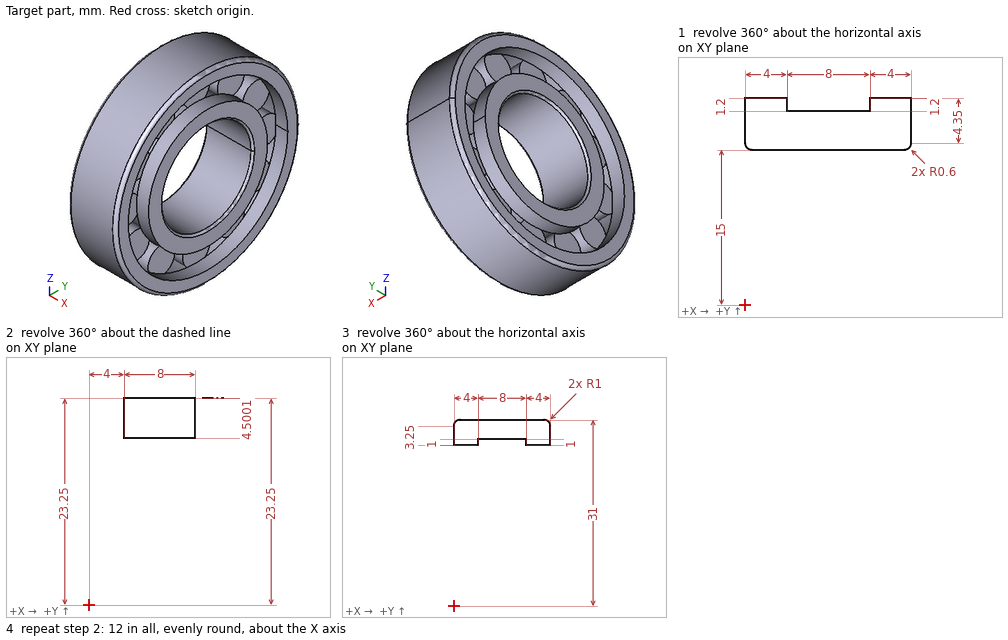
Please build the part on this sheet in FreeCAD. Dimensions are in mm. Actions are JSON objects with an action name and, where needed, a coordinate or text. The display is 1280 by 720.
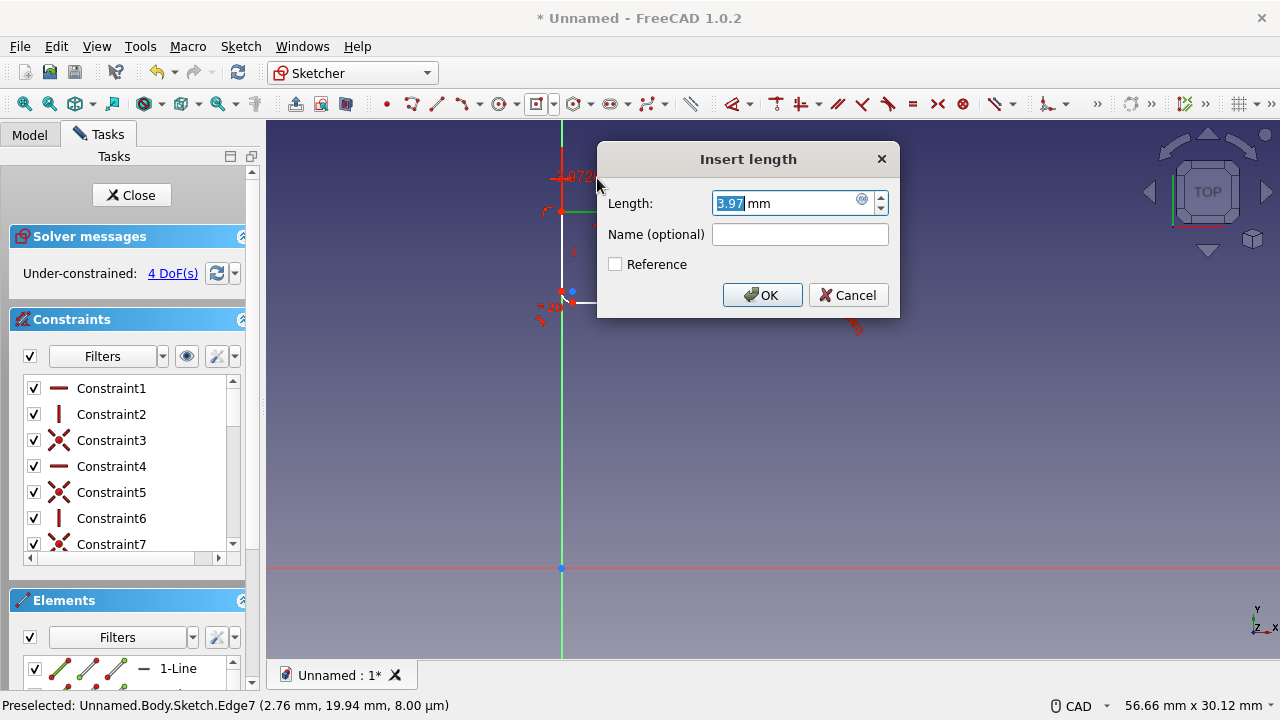
{"action": "type", "text": "4"}
{"action": "key", "text": "Return"}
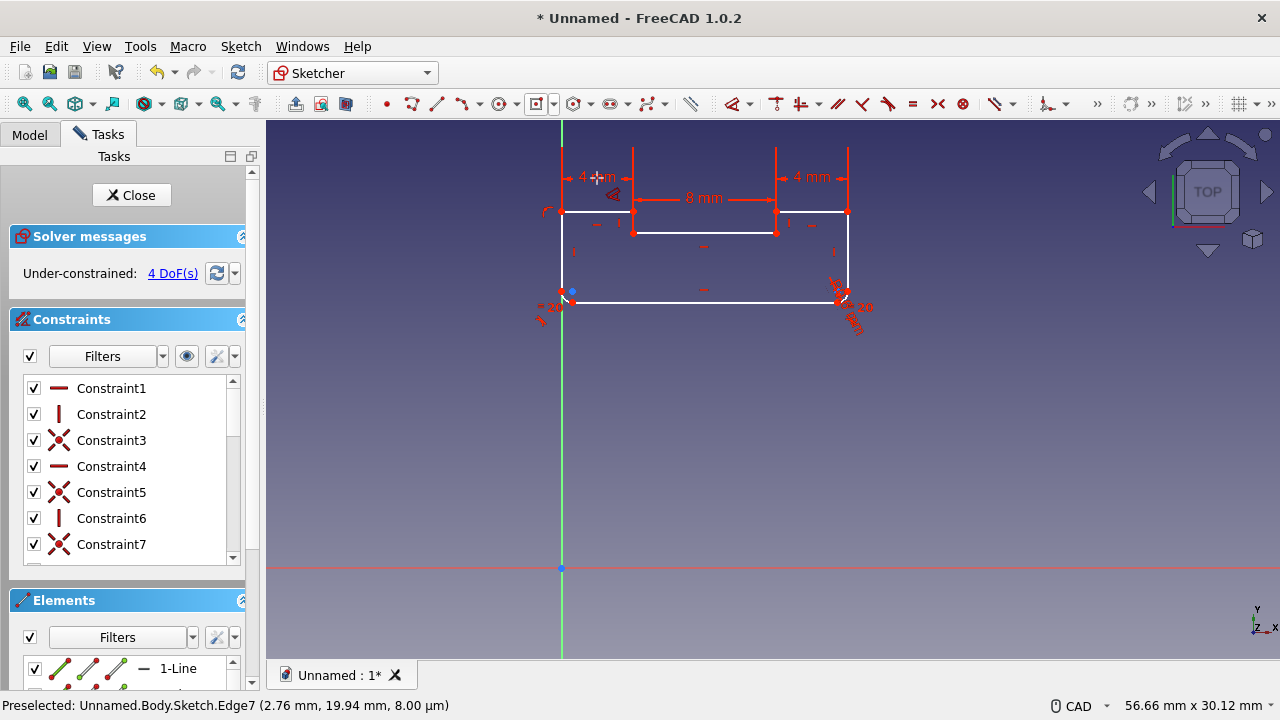
{"action": "scroll", "coordinate": [776, 223], "scroll_direction": "up", "scroll_amount": 4}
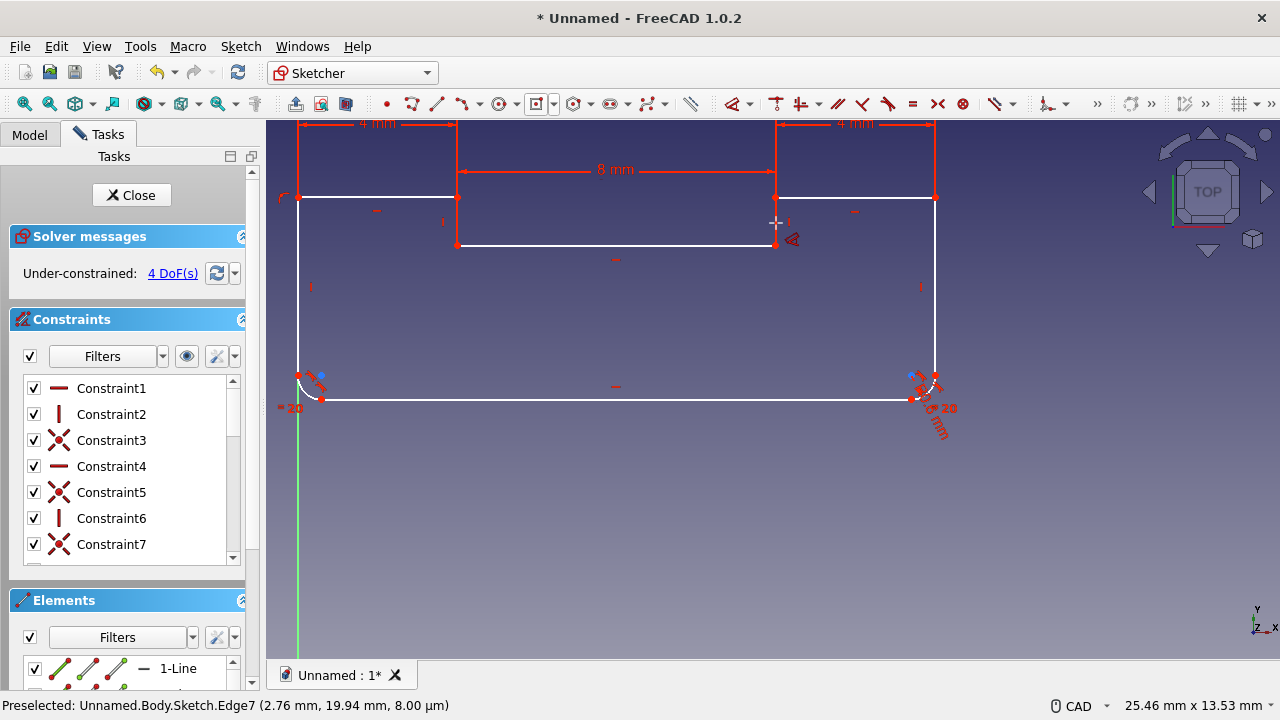
{"action": "left_click", "coordinate": [776, 222]}
{"action": "left_click", "coordinate": [810, 222]}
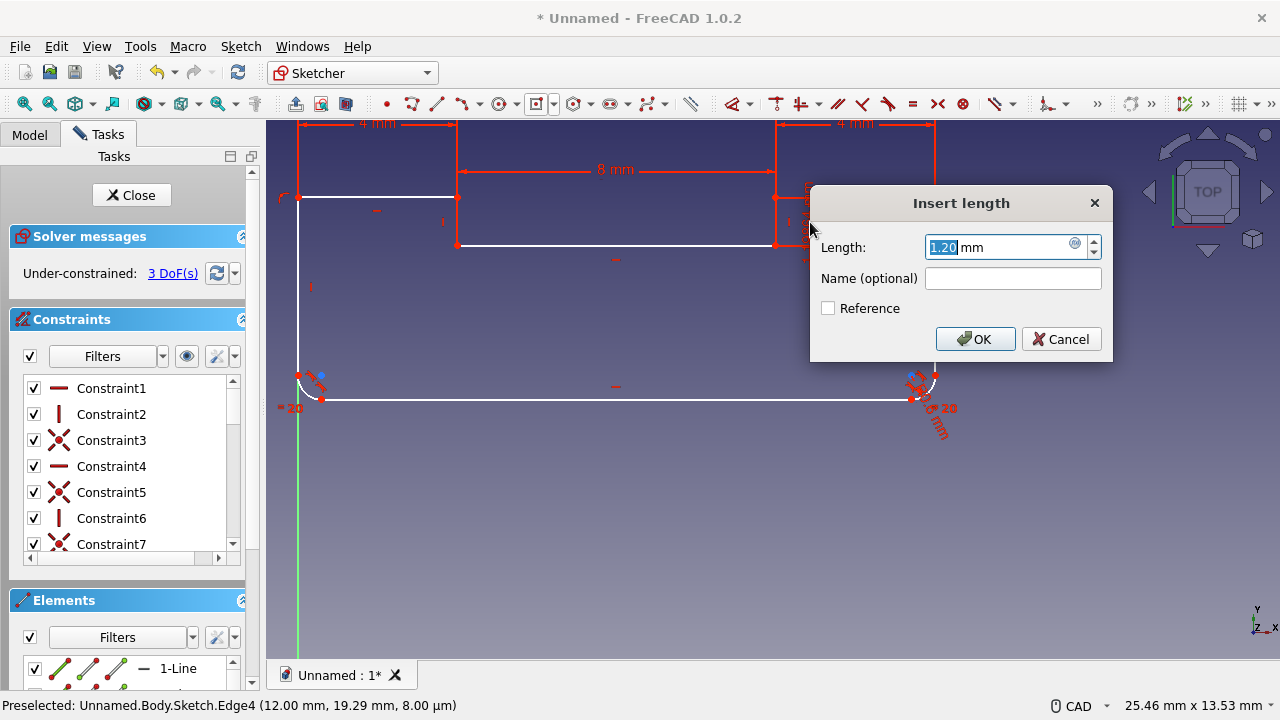
{"action": "type", "text": "1.2"}
{"action": "key", "text": "Return"}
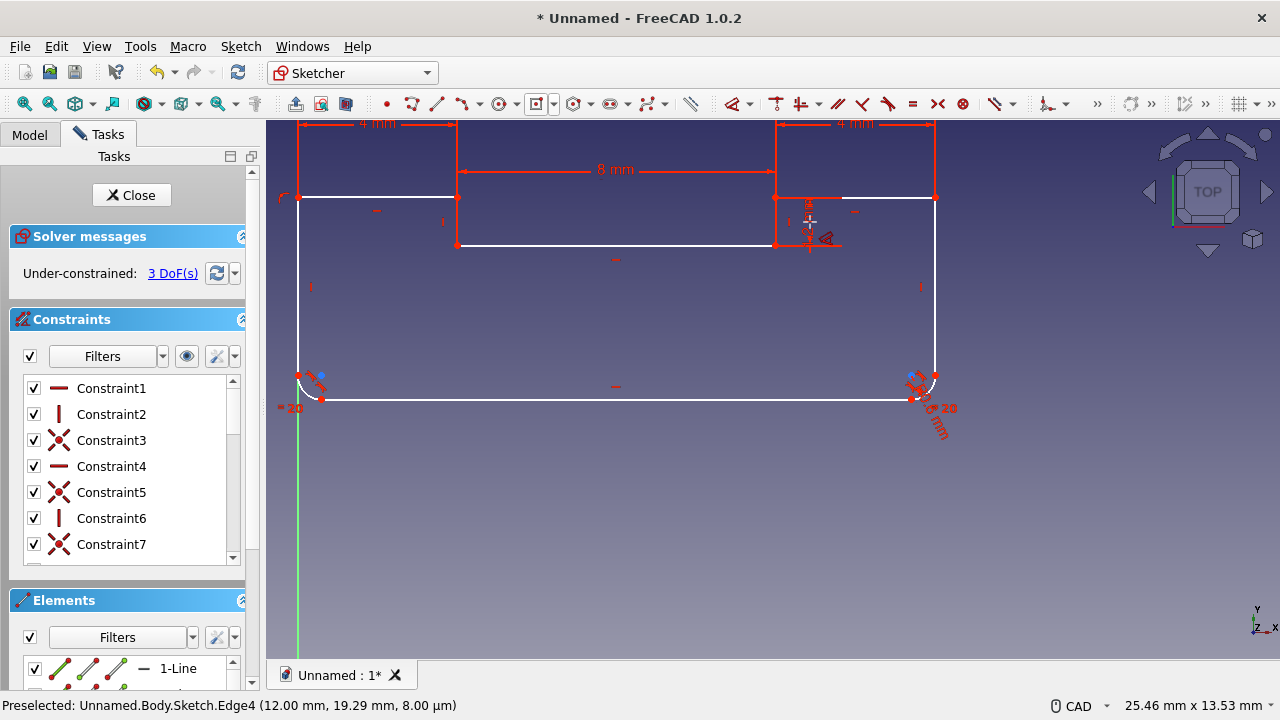
{"action": "left_click", "coordinate": [457, 231]}
{"action": "left_click", "coordinate": [423, 221]}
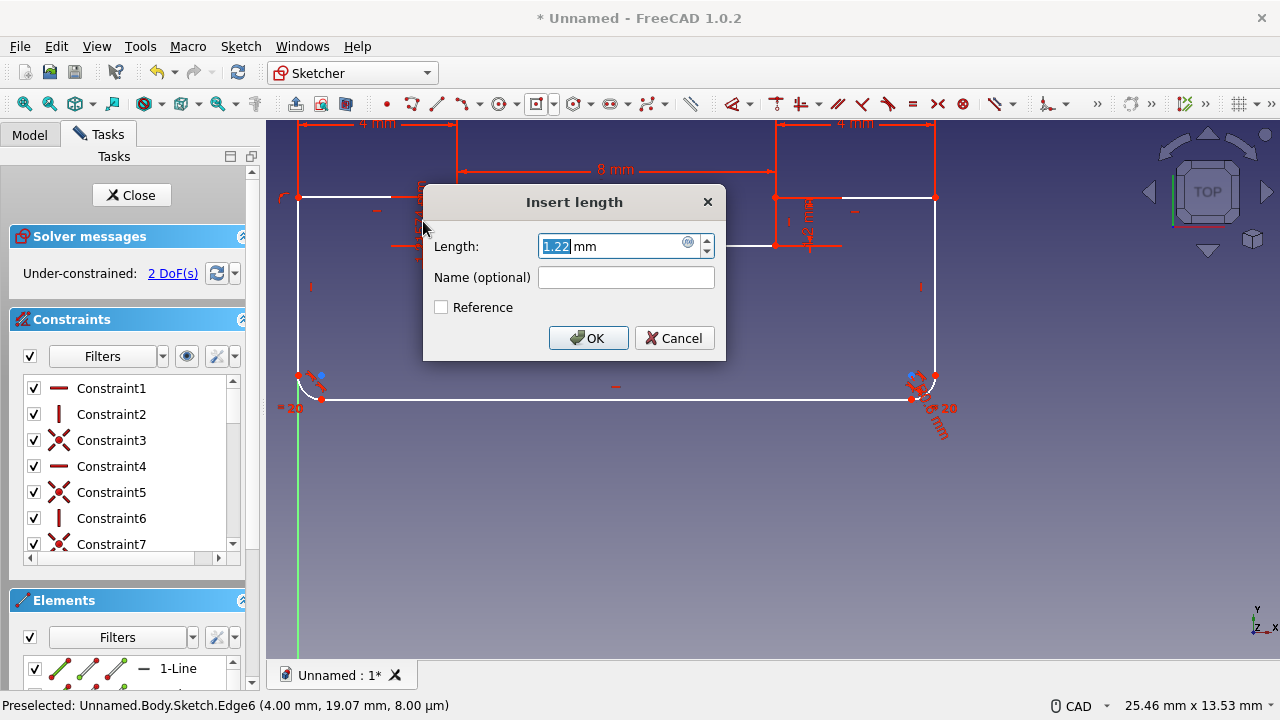
{"action": "type", "text": "1.2"}
{"action": "key", "text": "Return"}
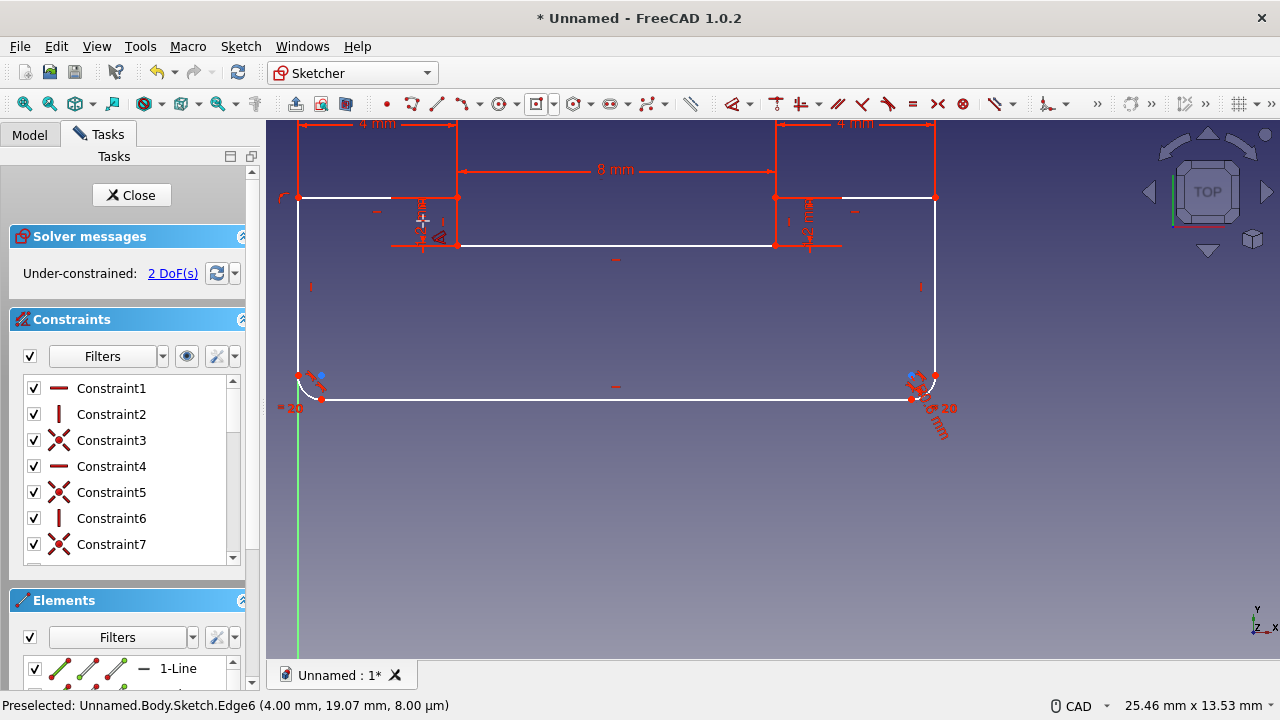
{"action": "left_click", "coordinate": [322, 400]}
{"action": "left_click", "coordinate": [356, 515]}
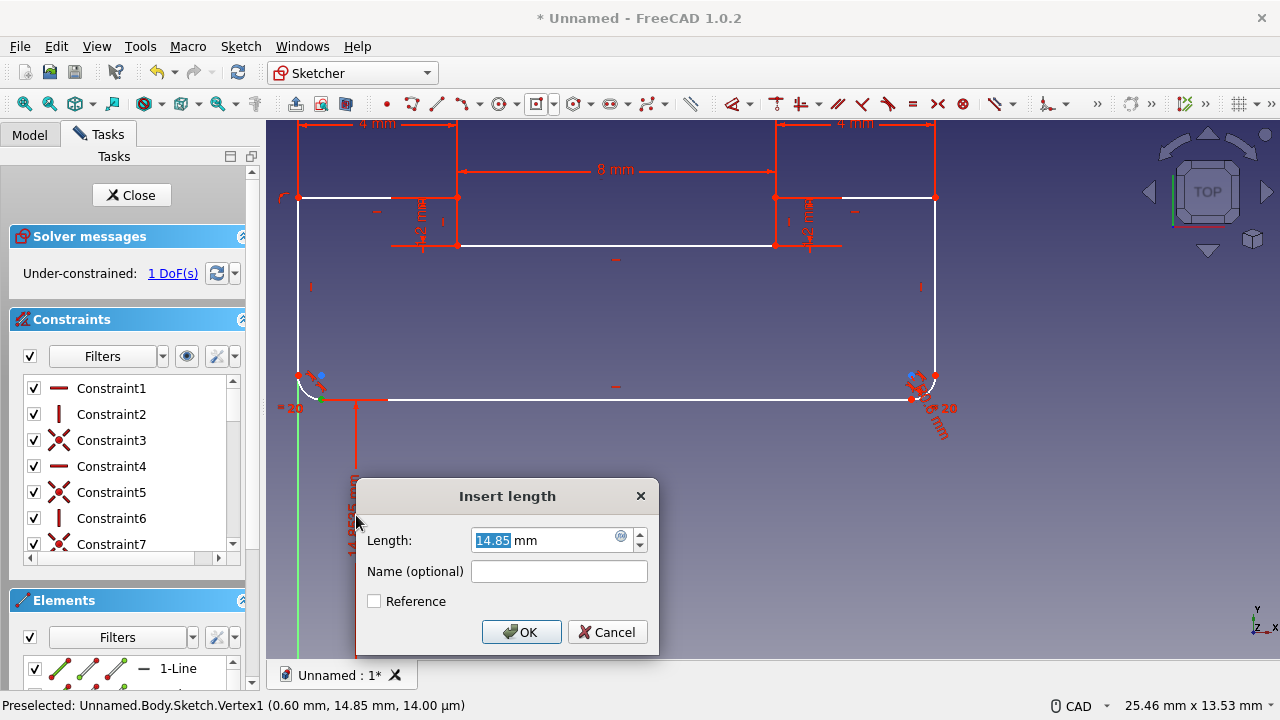
{"action": "type", "text": "15"}
{"action": "key", "text": "Return"}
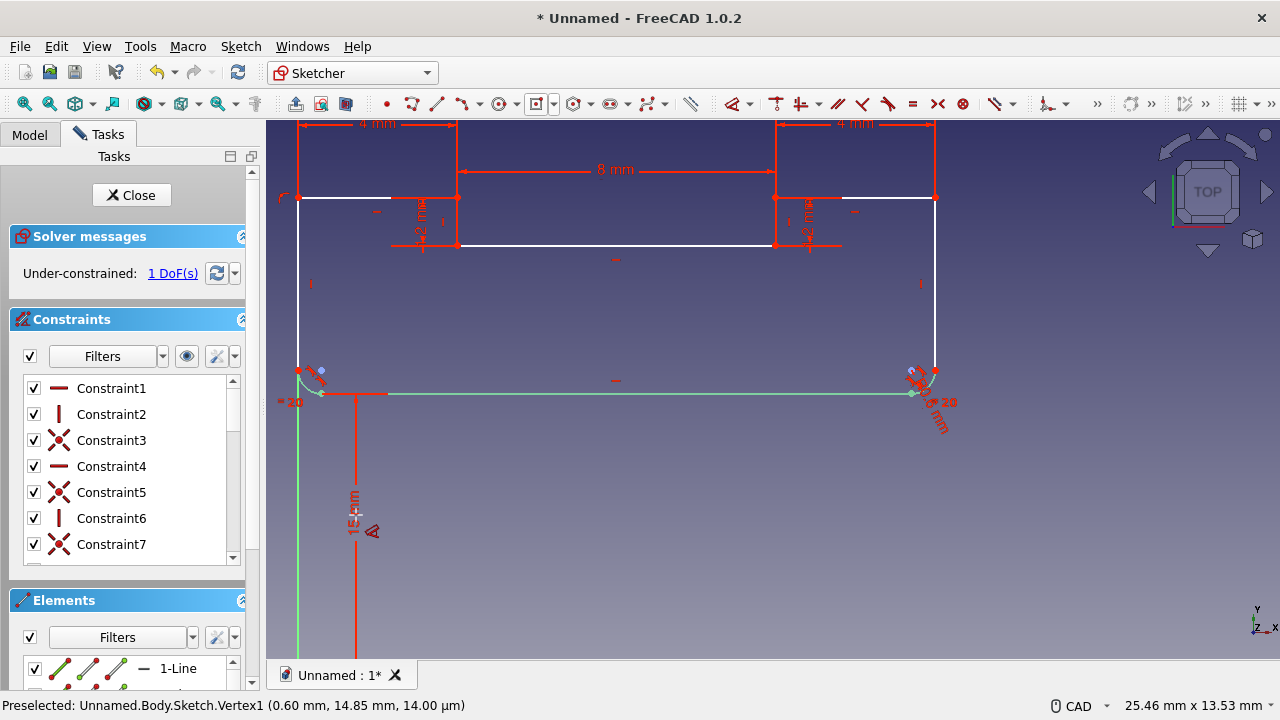
{"action": "left_click", "coordinate": [935, 318]}
{"action": "left_click", "coordinate": [969, 284]}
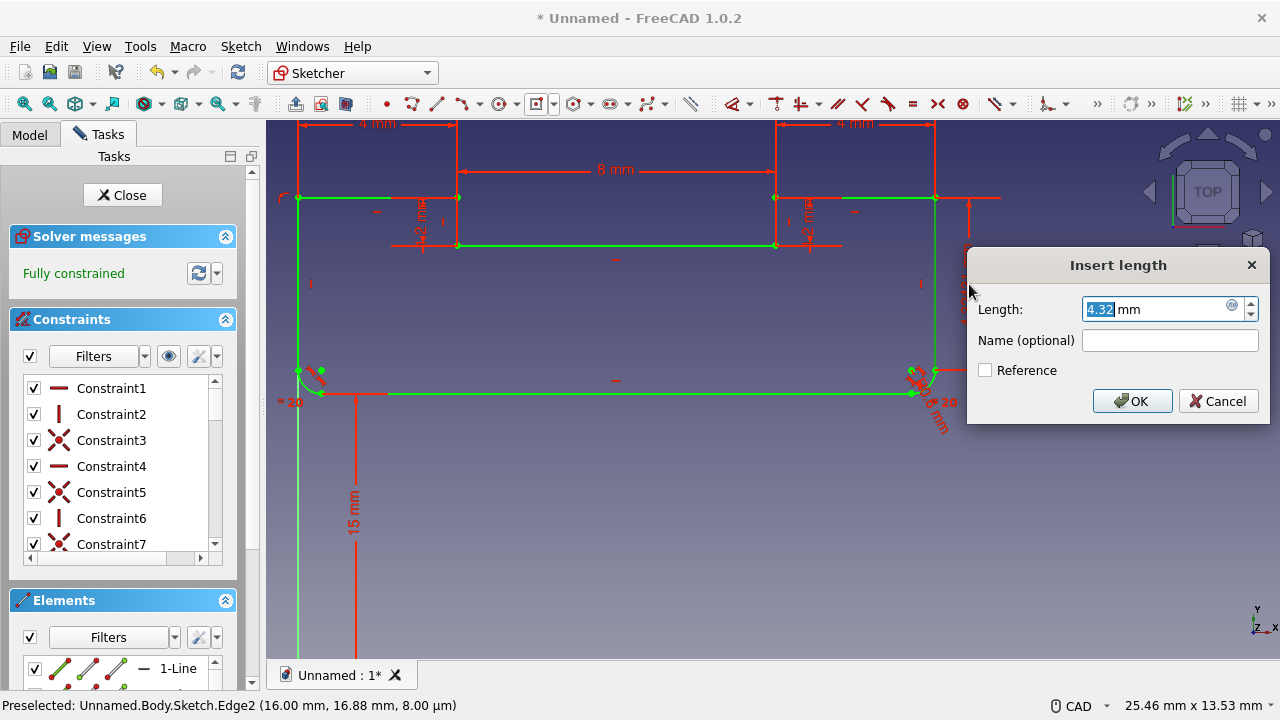
{"action": "type", "text": "4.35"}
{"action": "key", "text": "Return"}
{"action": "key", "text": "Escape"}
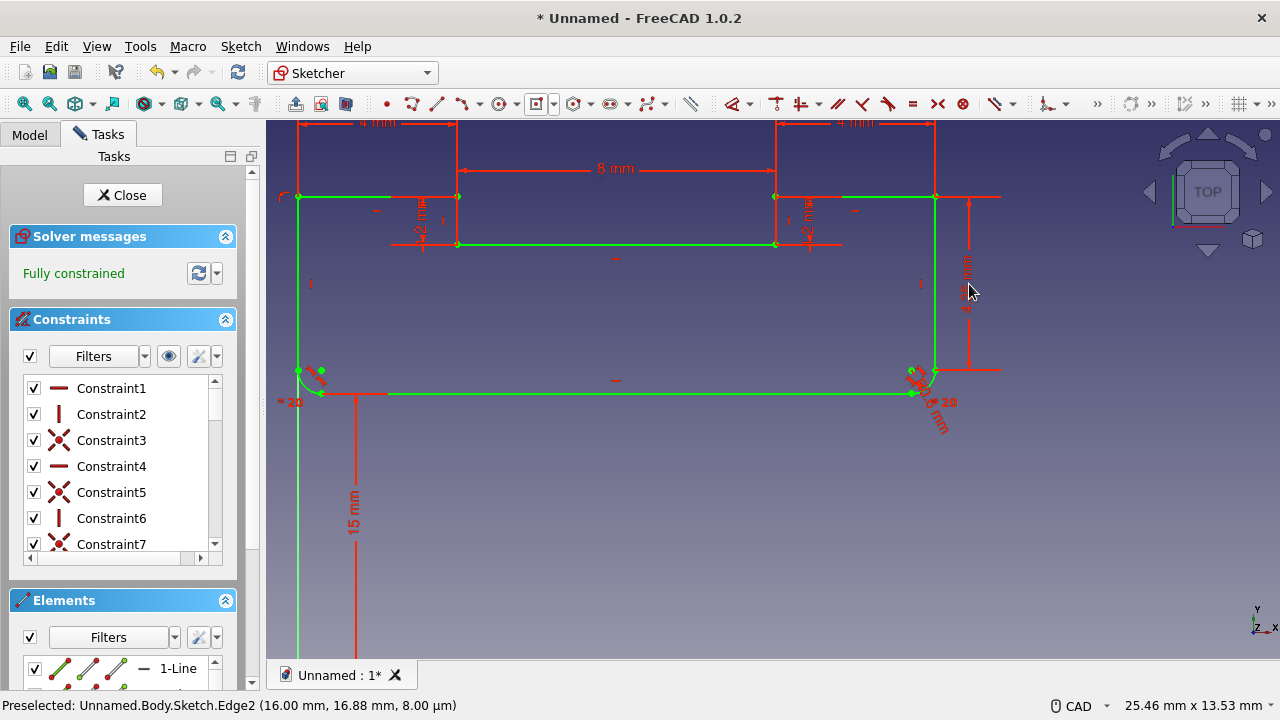
{"action": "left_click", "coordinate": [123, 195]}